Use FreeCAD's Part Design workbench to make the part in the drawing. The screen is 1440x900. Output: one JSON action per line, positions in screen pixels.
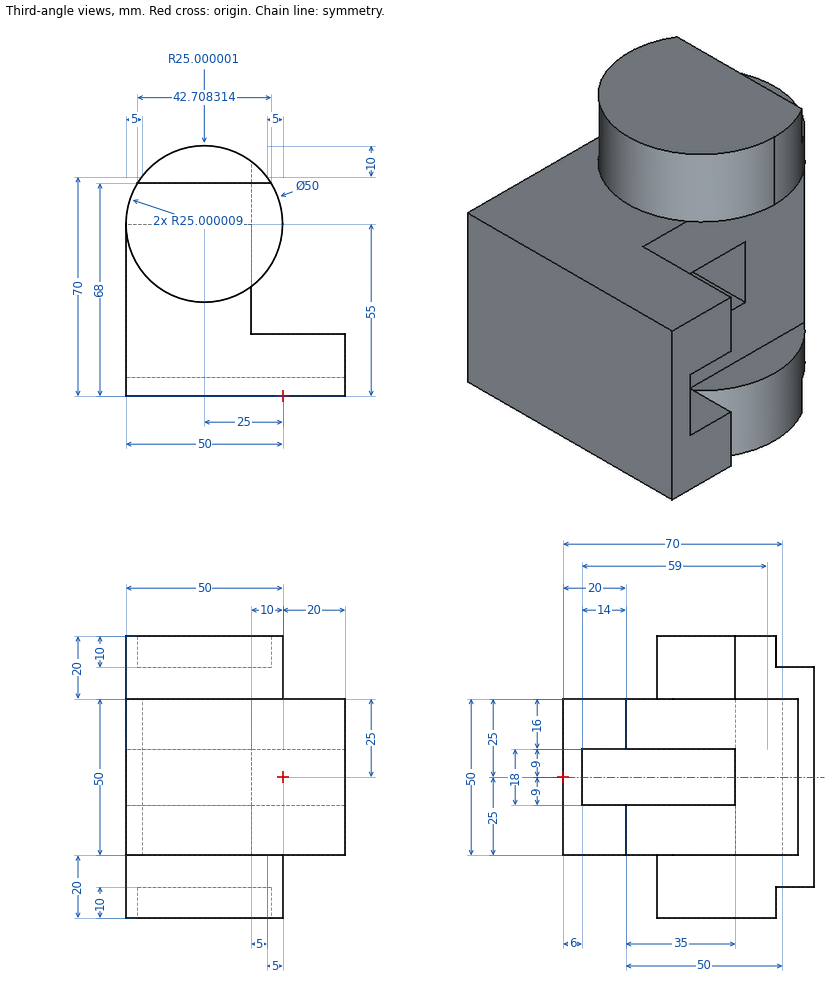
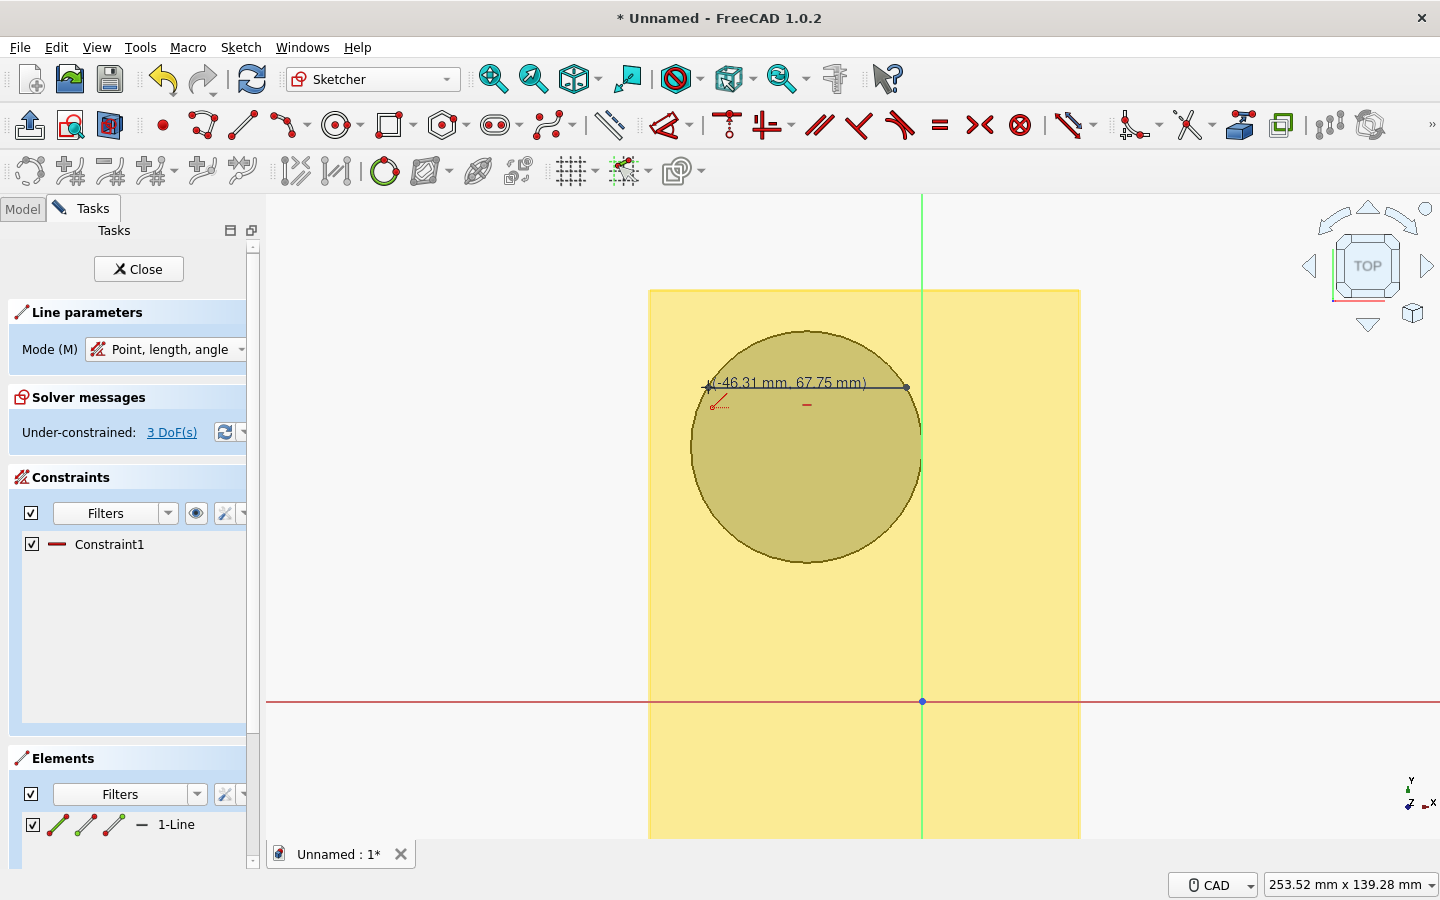
{"action": "left_click", "coordinate": [284, 126]}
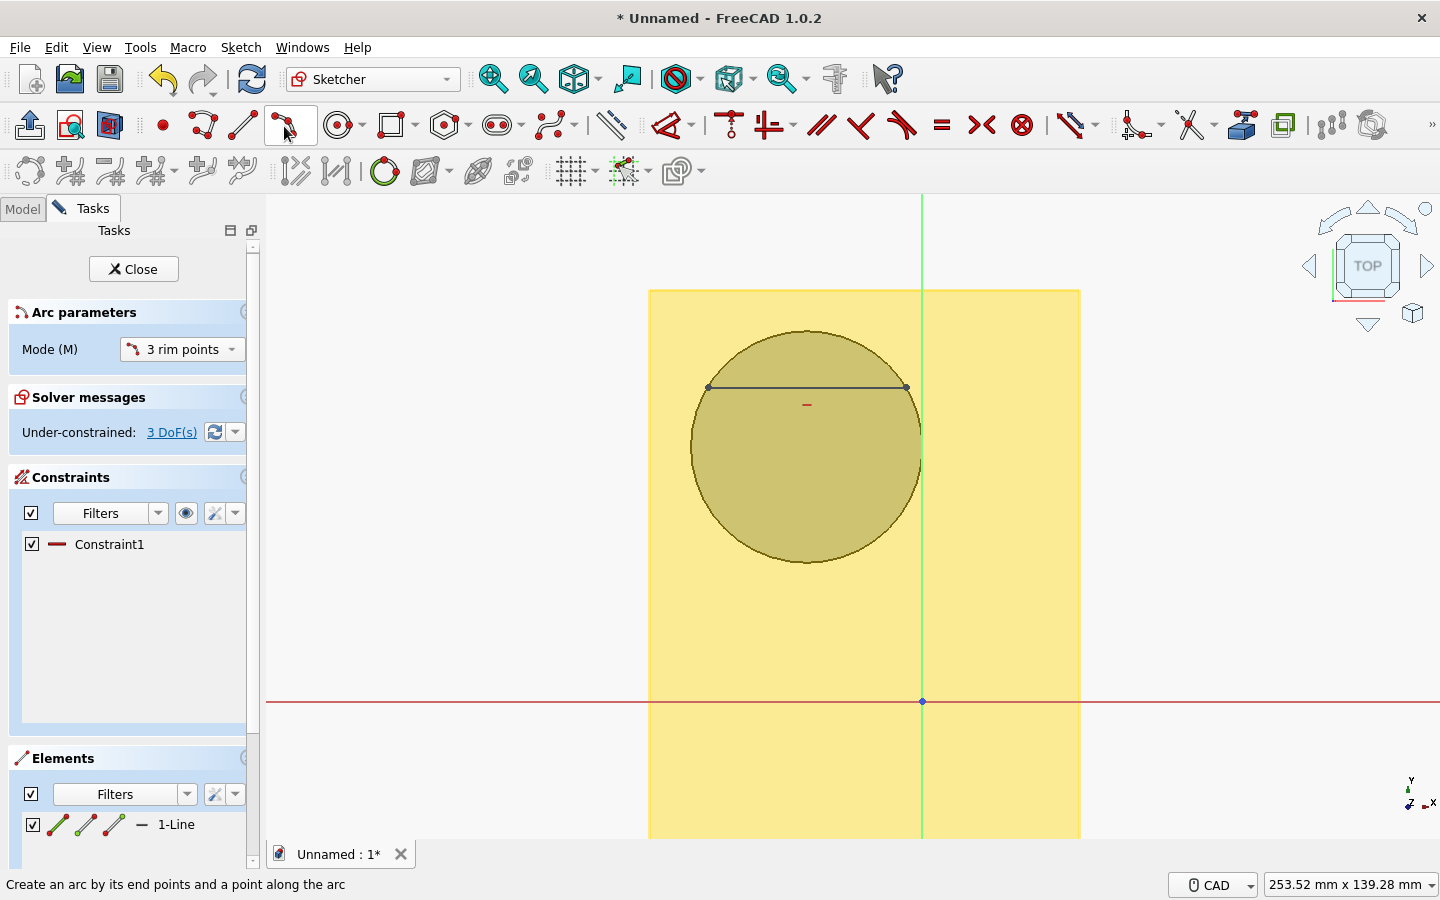
{"action": "left_click", "coordinate": [708, 388]}
{"action": "left_click", "coordinate": [906, 388]}
{"action": "left_click", "coordinate": [807, 331]}
{"action": "key", "text": "Escape"}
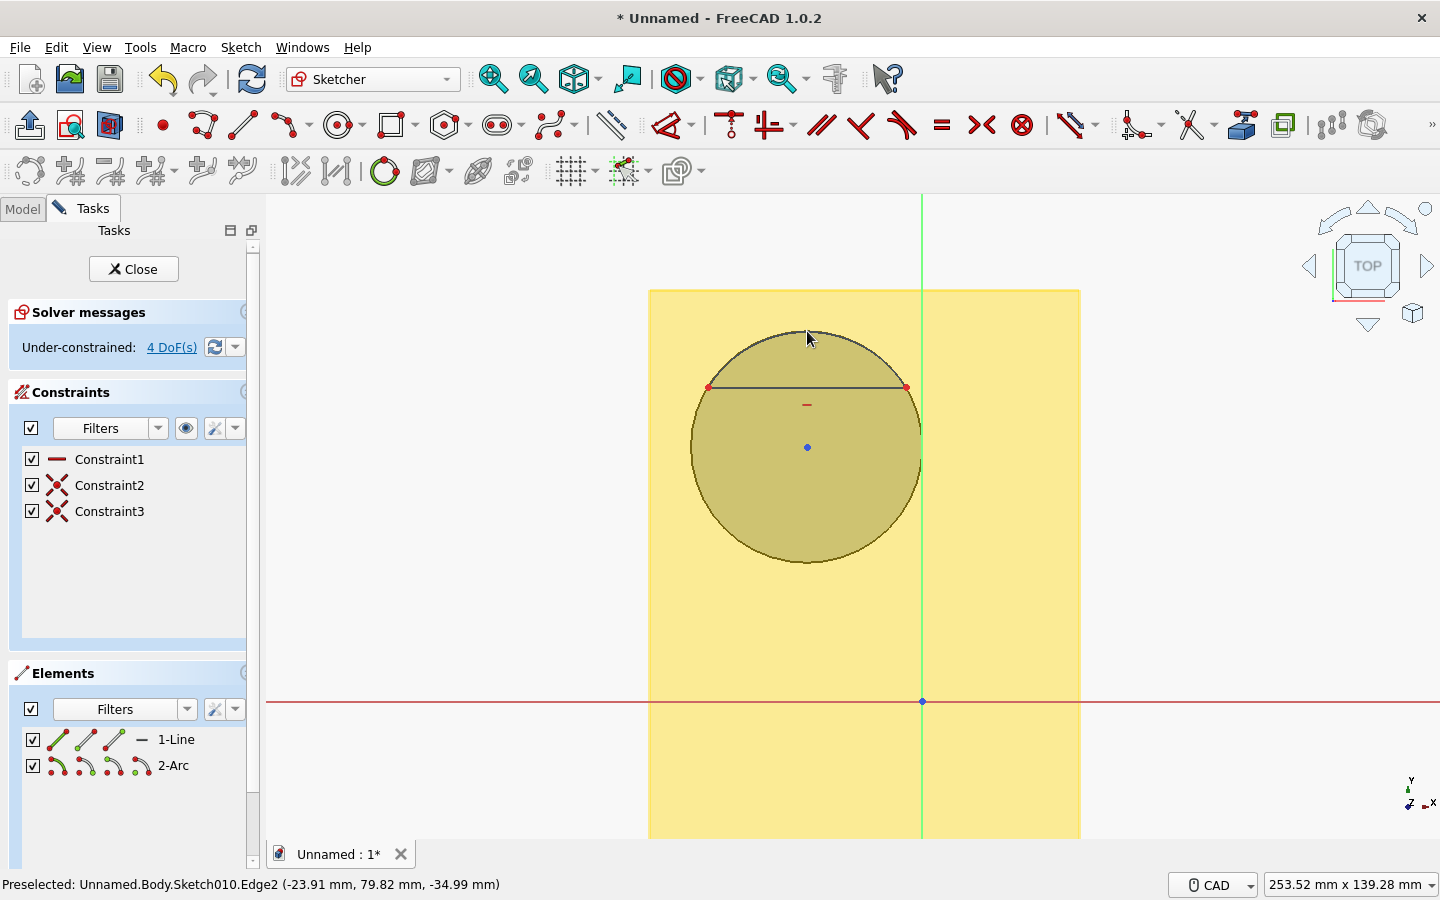
{"action": "left_click", "coordinate": [666, 126]}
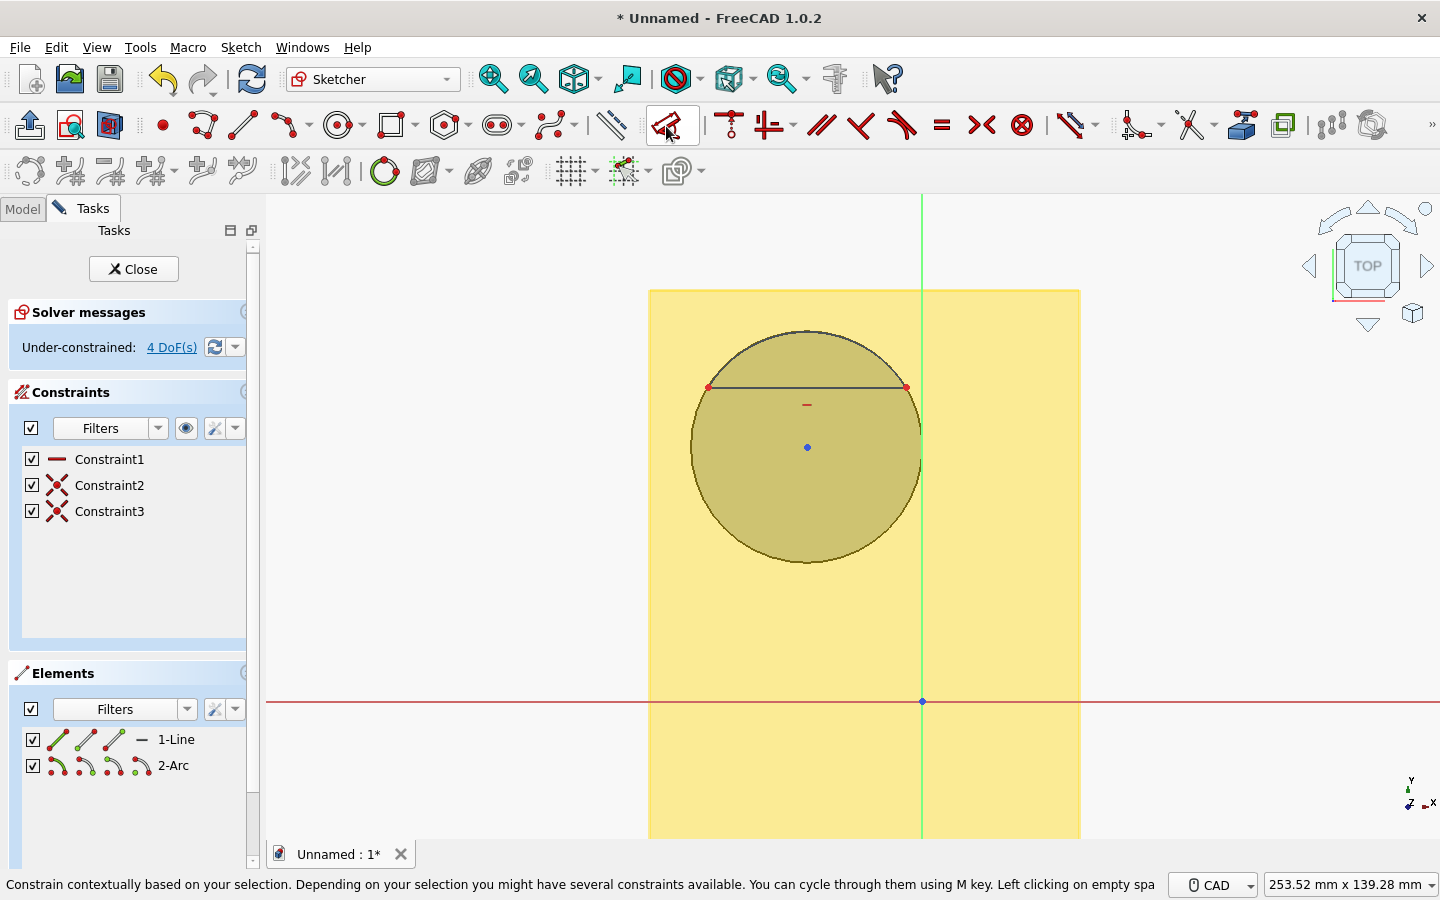
{"action": "left_click", "coordinate": [853, 342]}
{"action": "left_click", "coordinate": [866, 313]}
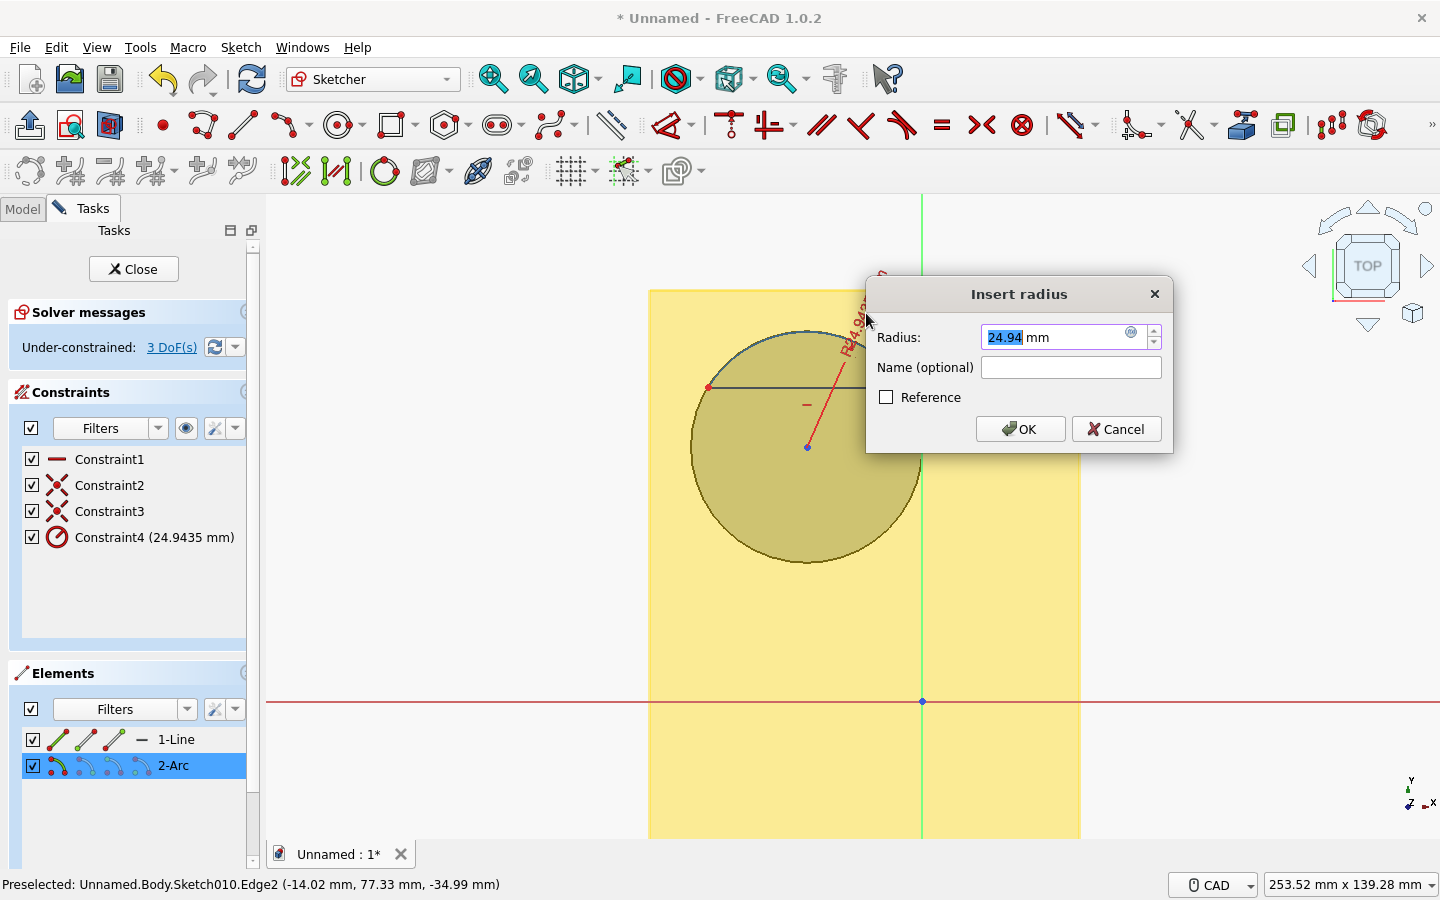
{"action": "type", "text": "25.000001"}
{"action": "key", "text": "Return"}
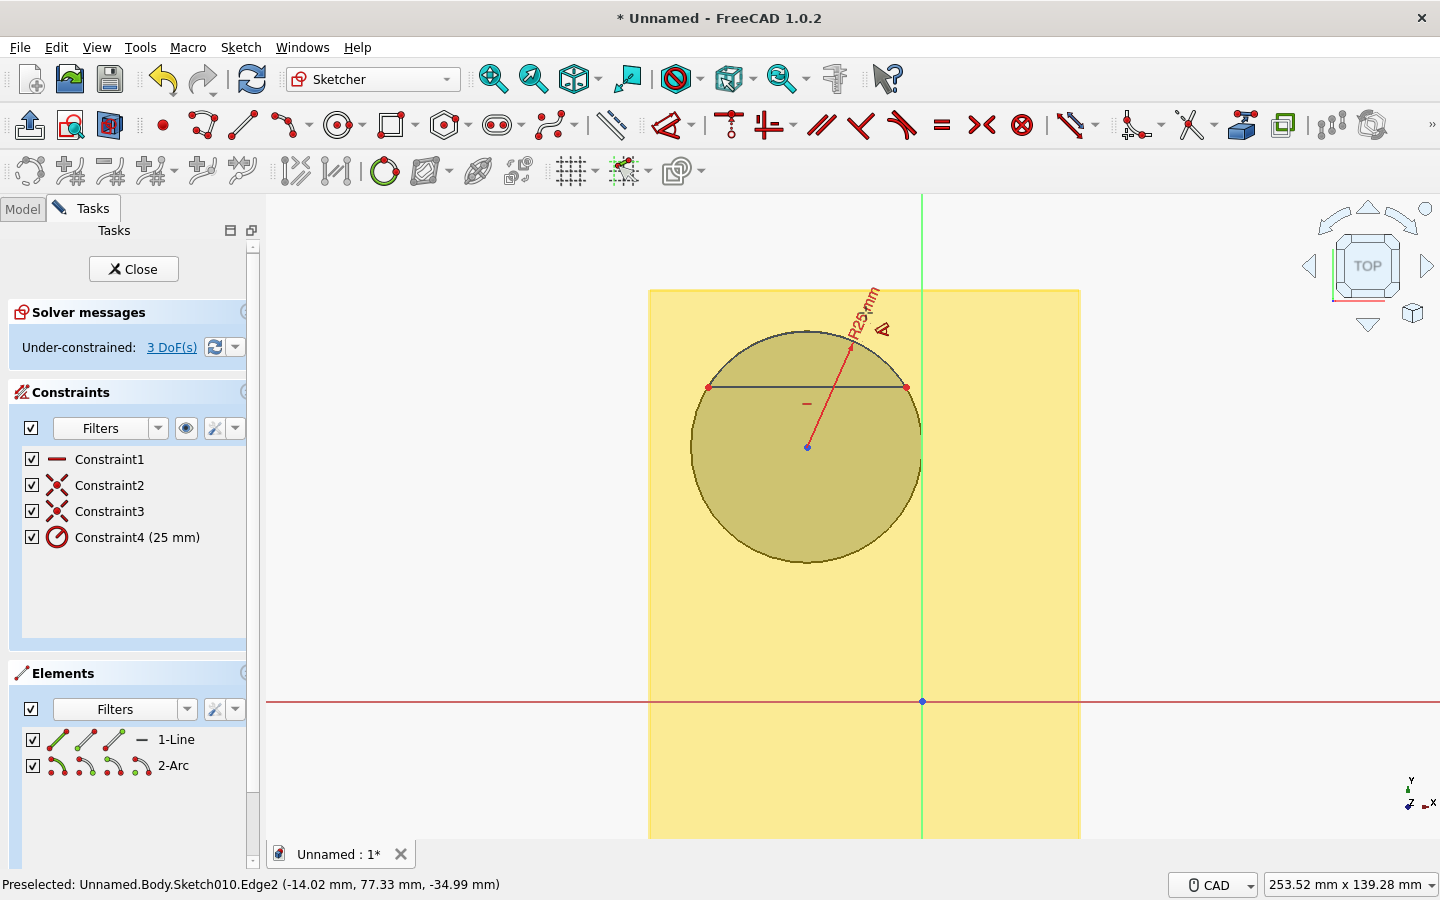
{"action": "left_click", "coordinate": [906, 387]}
{"action": "left_click", "coordinate": [956, 545]}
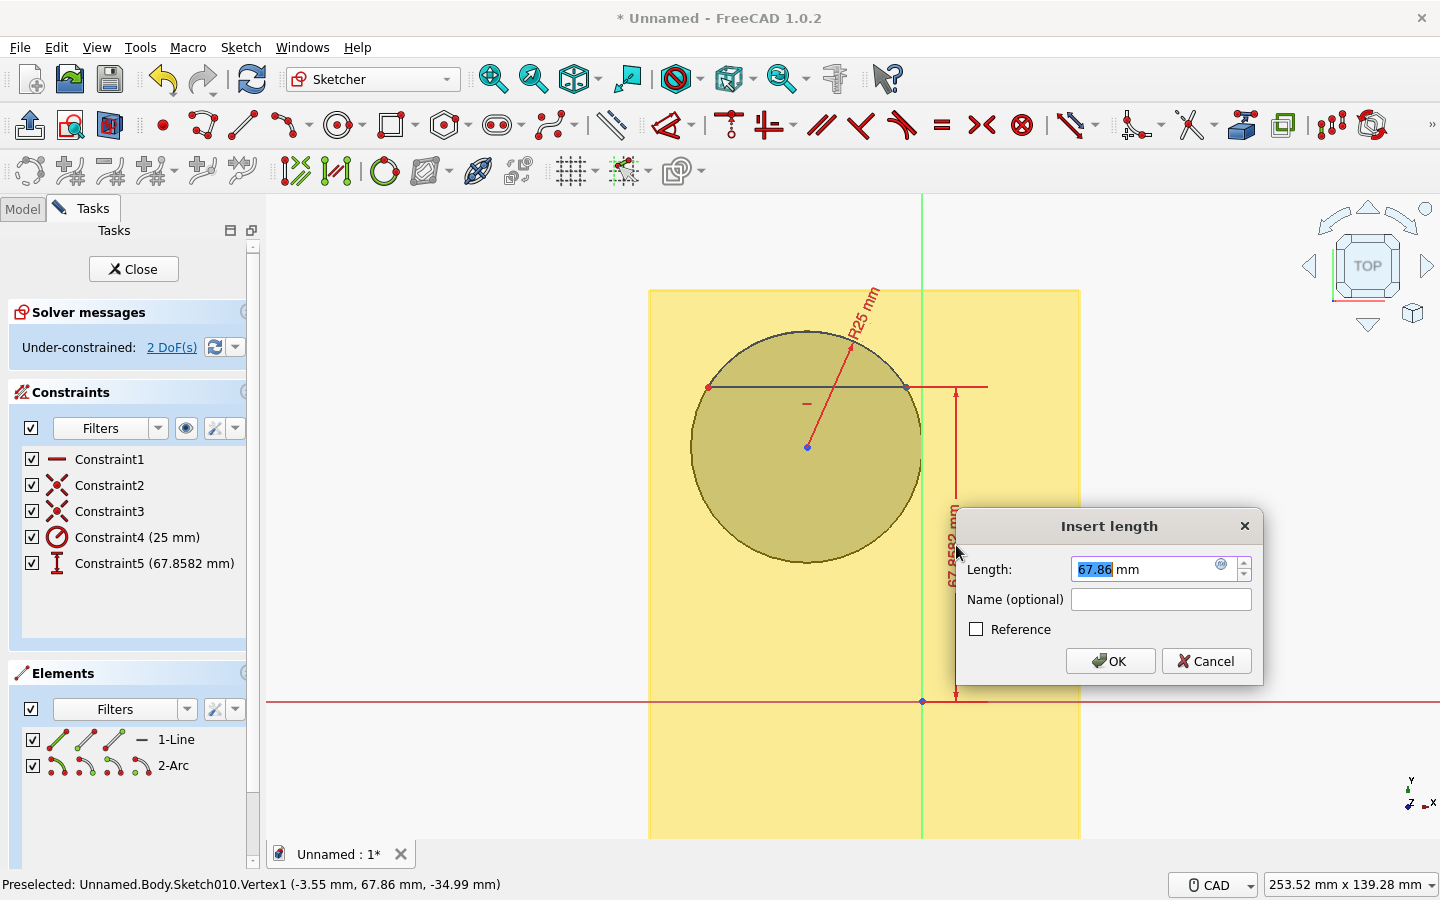
{"action": "type", "text": "68"}
{"action": "key", "text": "Return"}